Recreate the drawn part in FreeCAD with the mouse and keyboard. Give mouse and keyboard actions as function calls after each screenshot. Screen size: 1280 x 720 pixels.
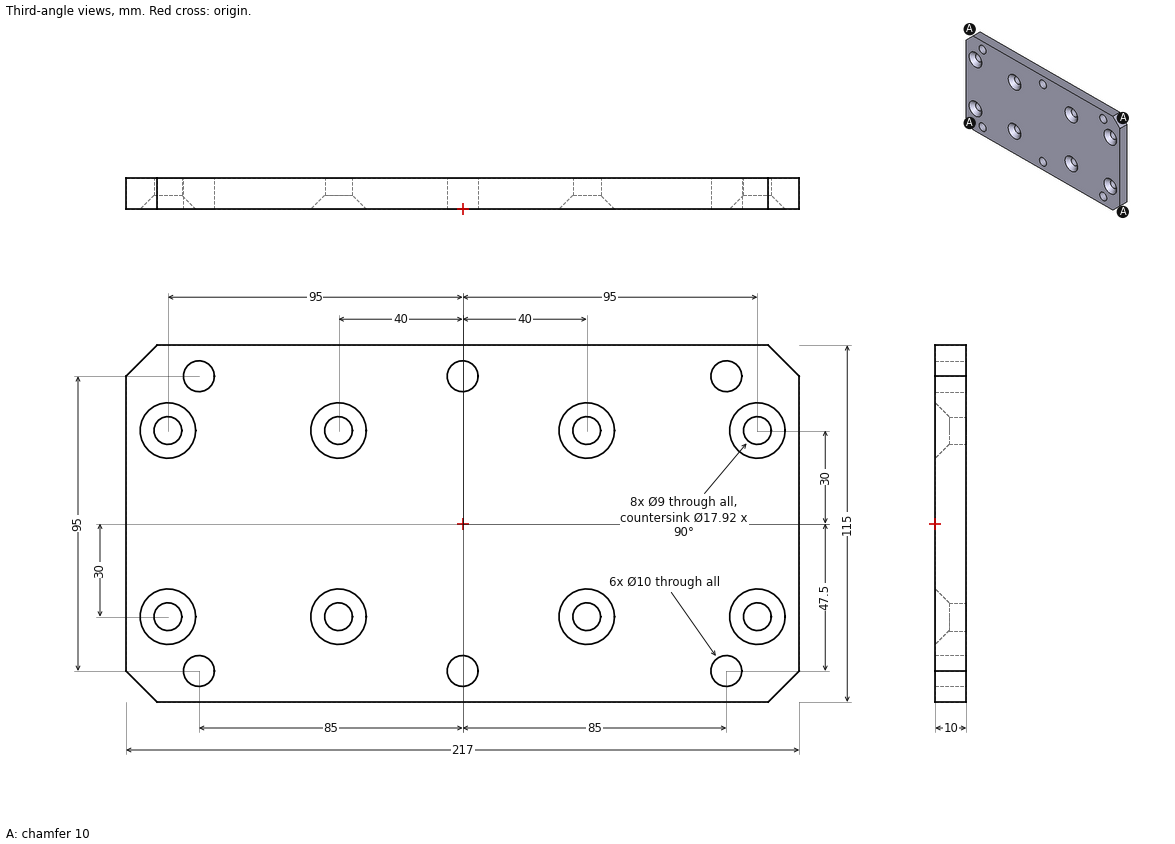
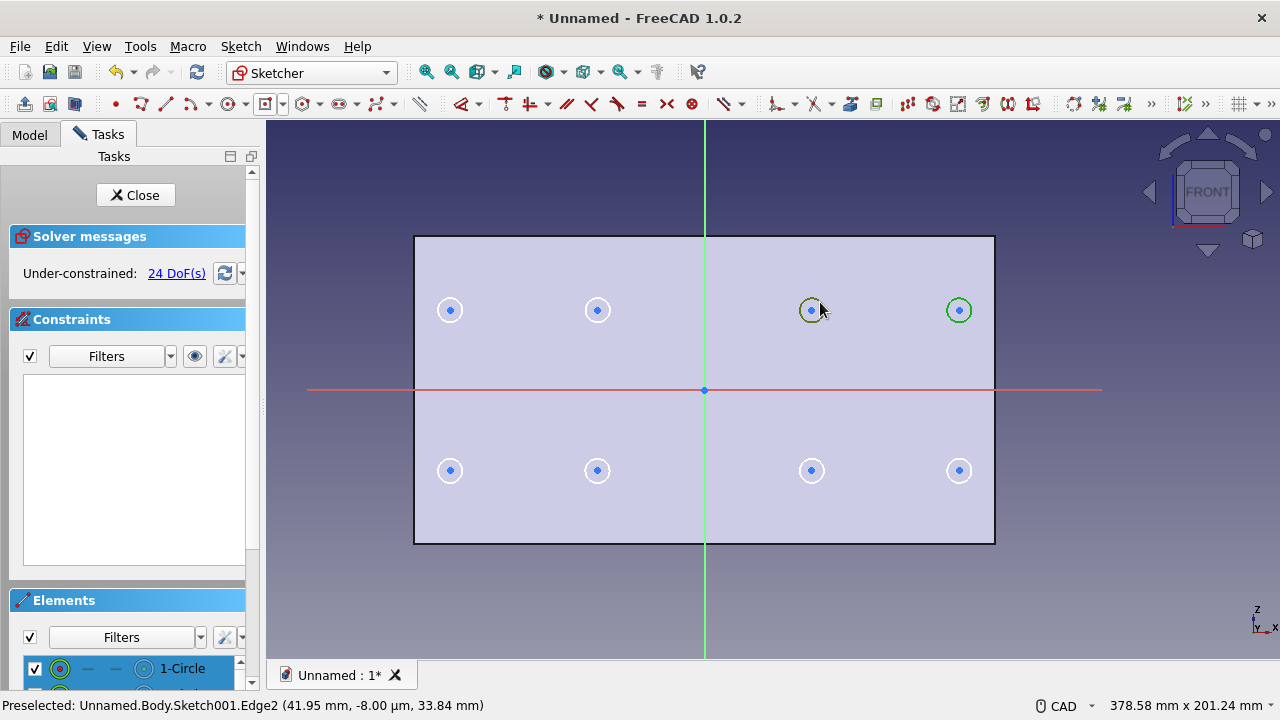
click(606, 302)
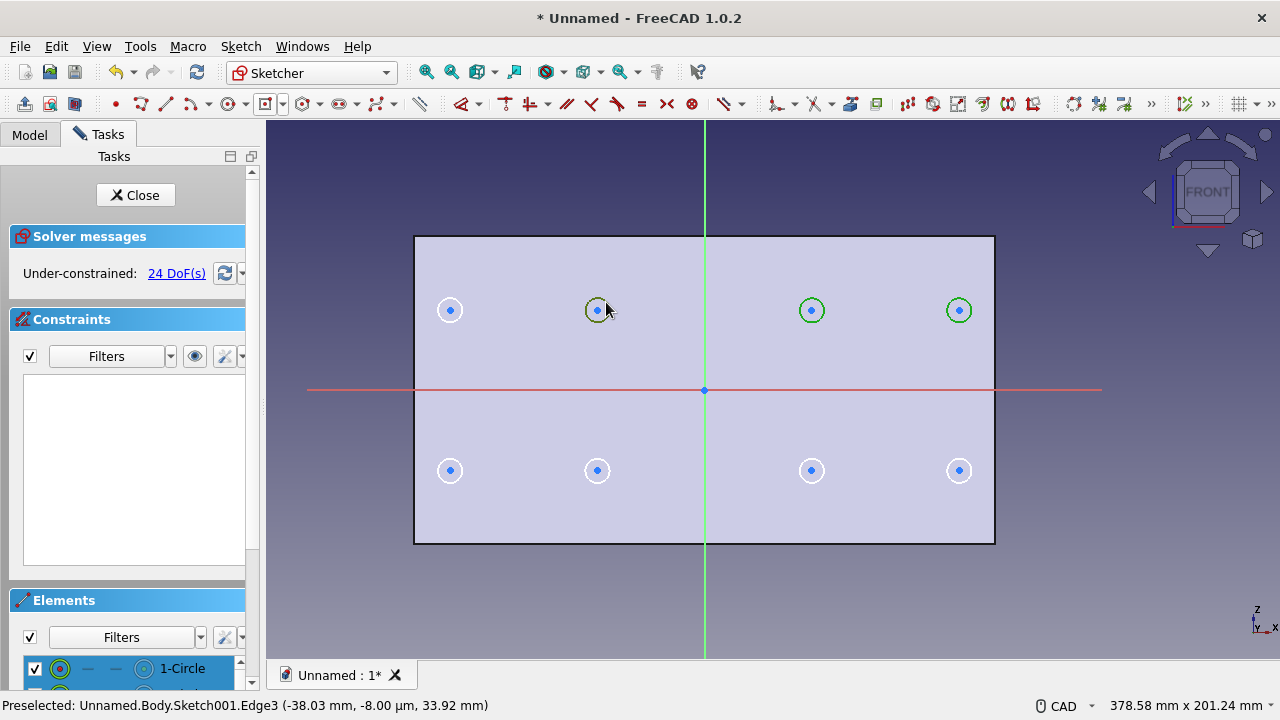
click(459, 302)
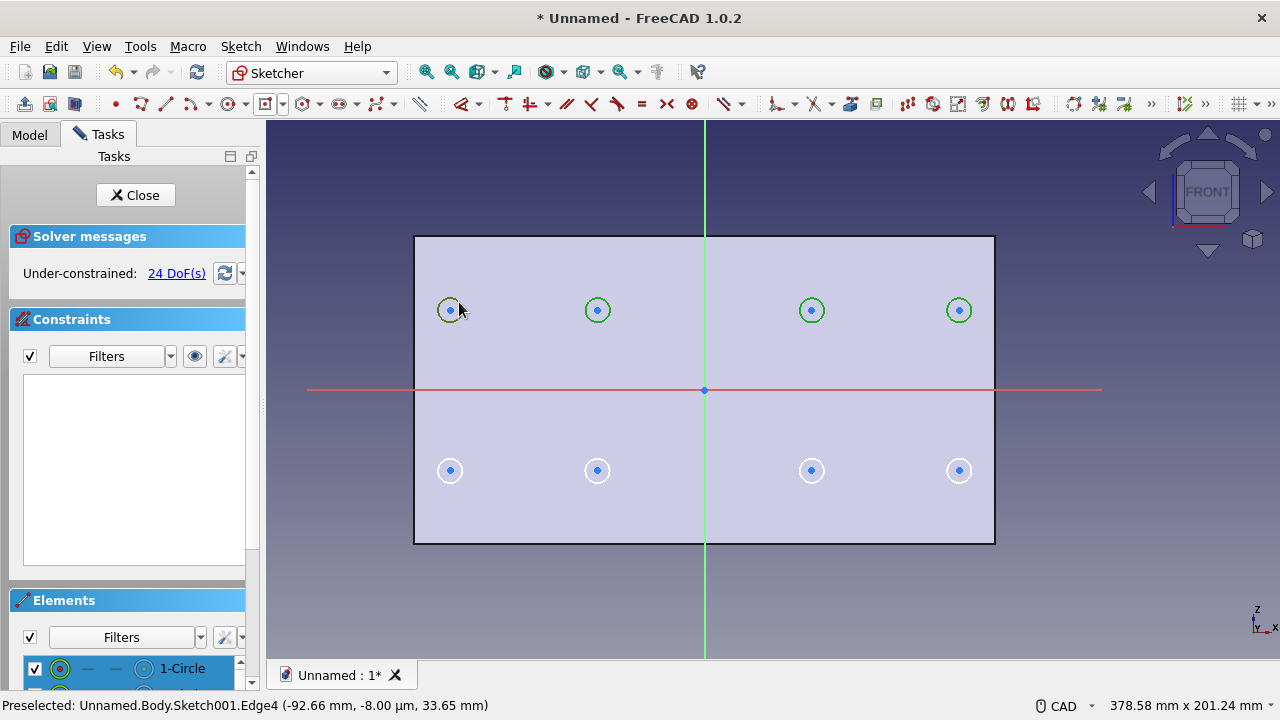
click(459, 462)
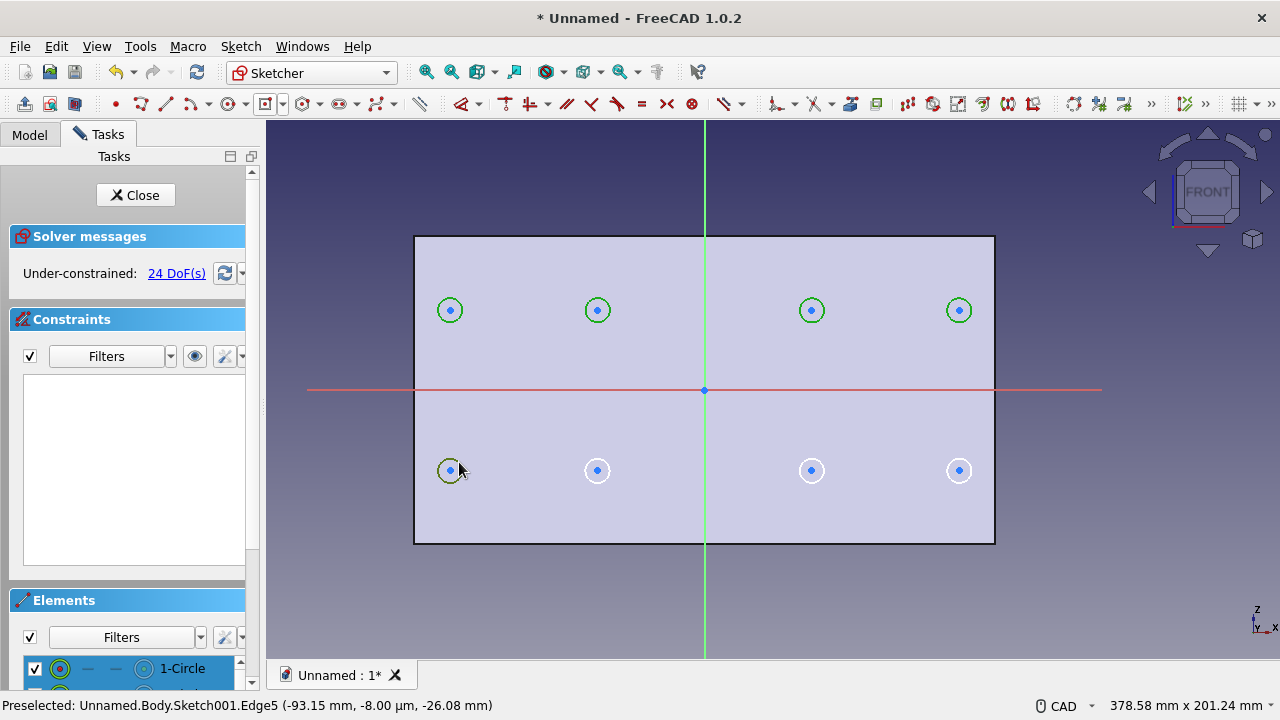
click(606, 462)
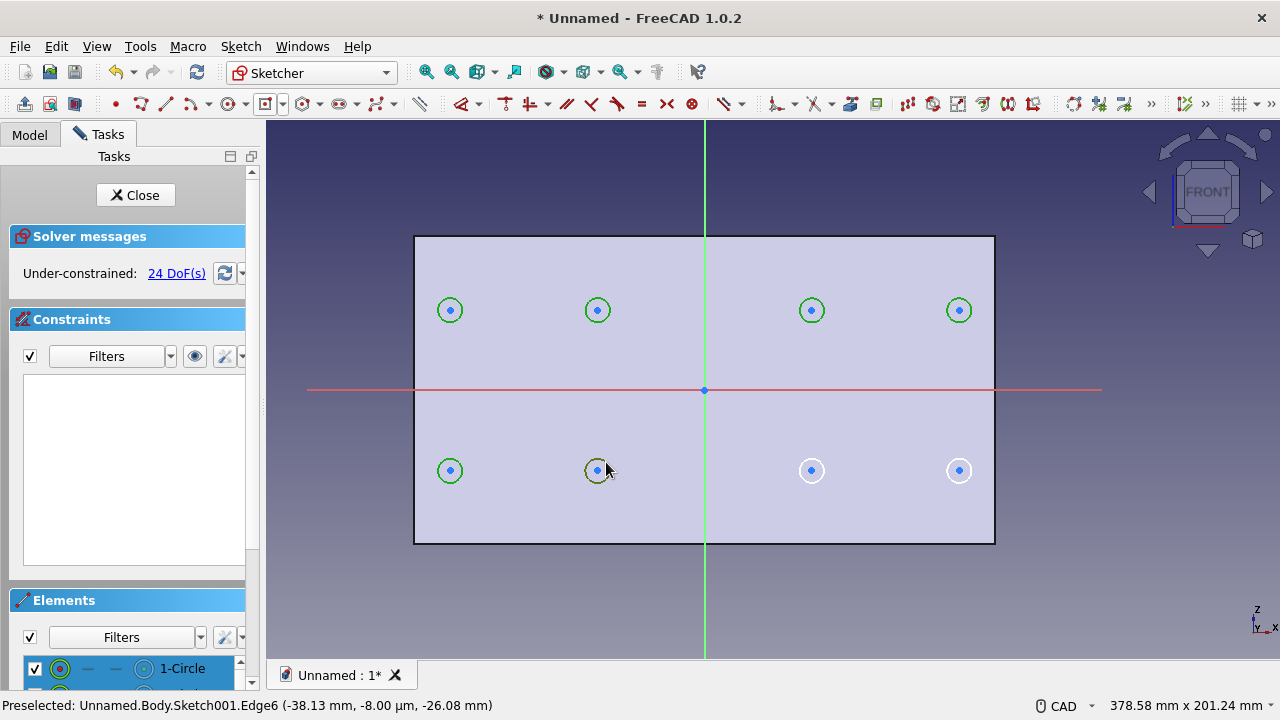
click(820, 462)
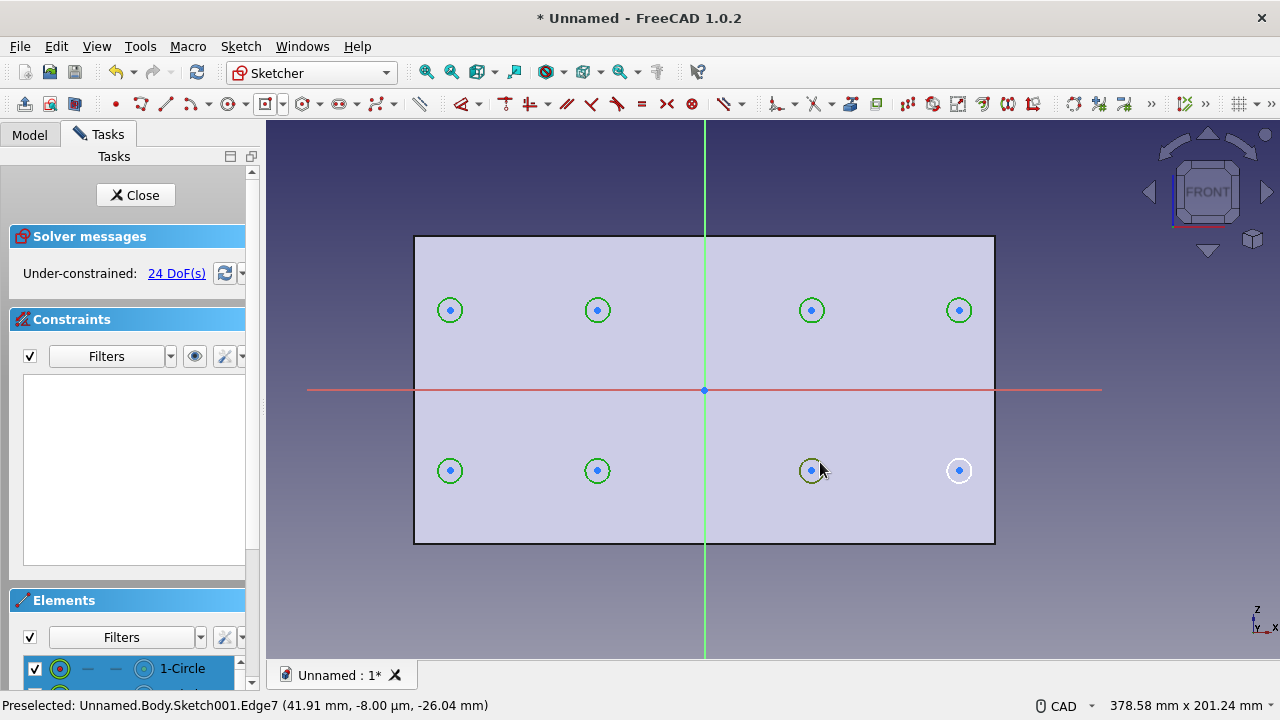
click(968, 462)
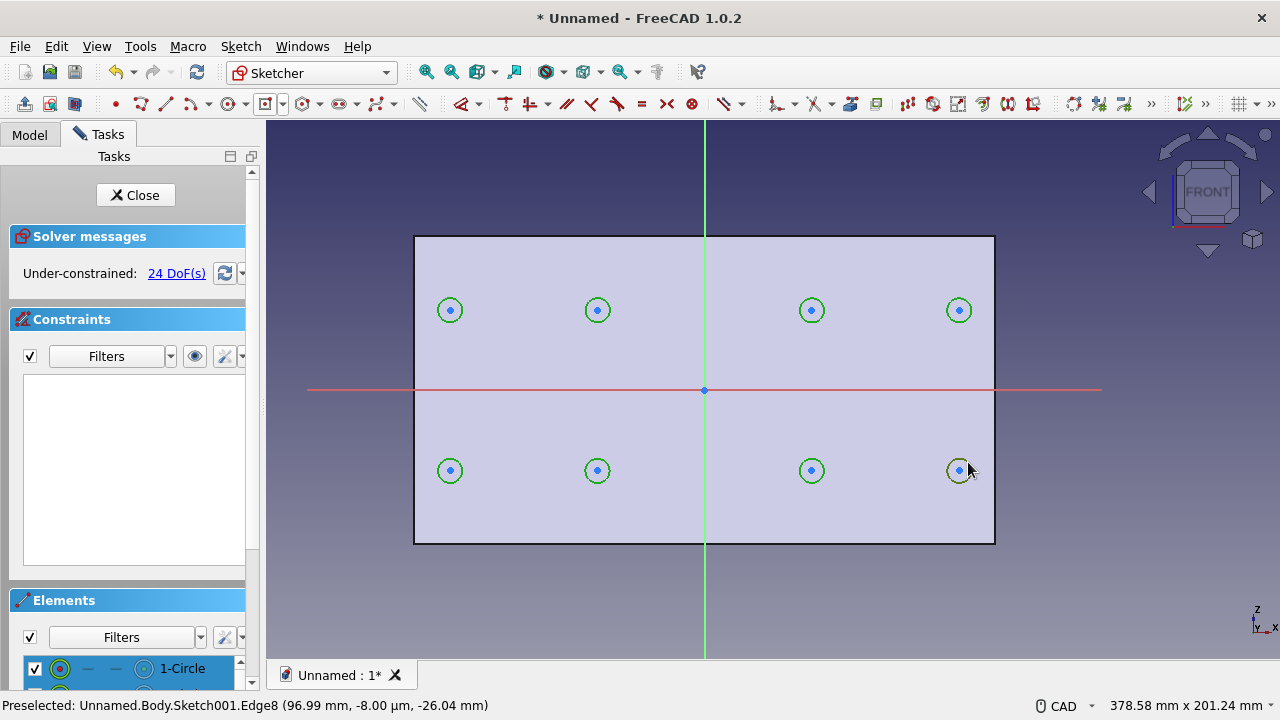
click(642, 104)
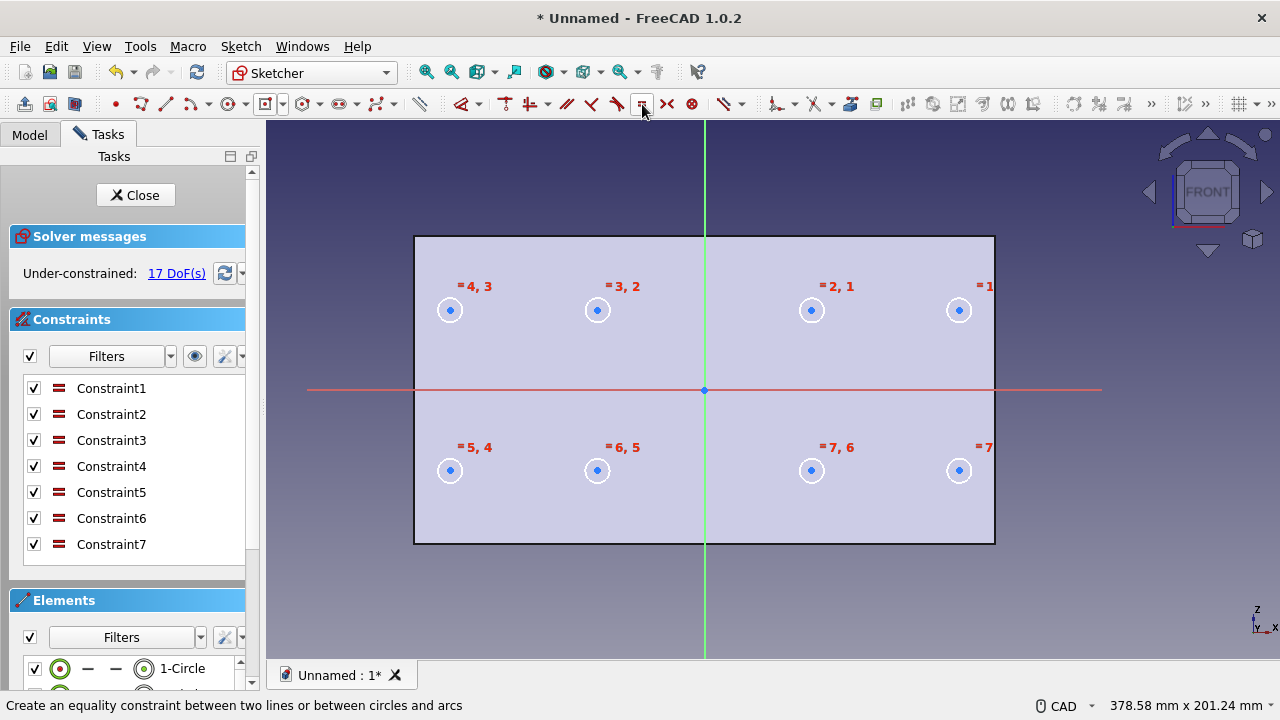
click(460, 104)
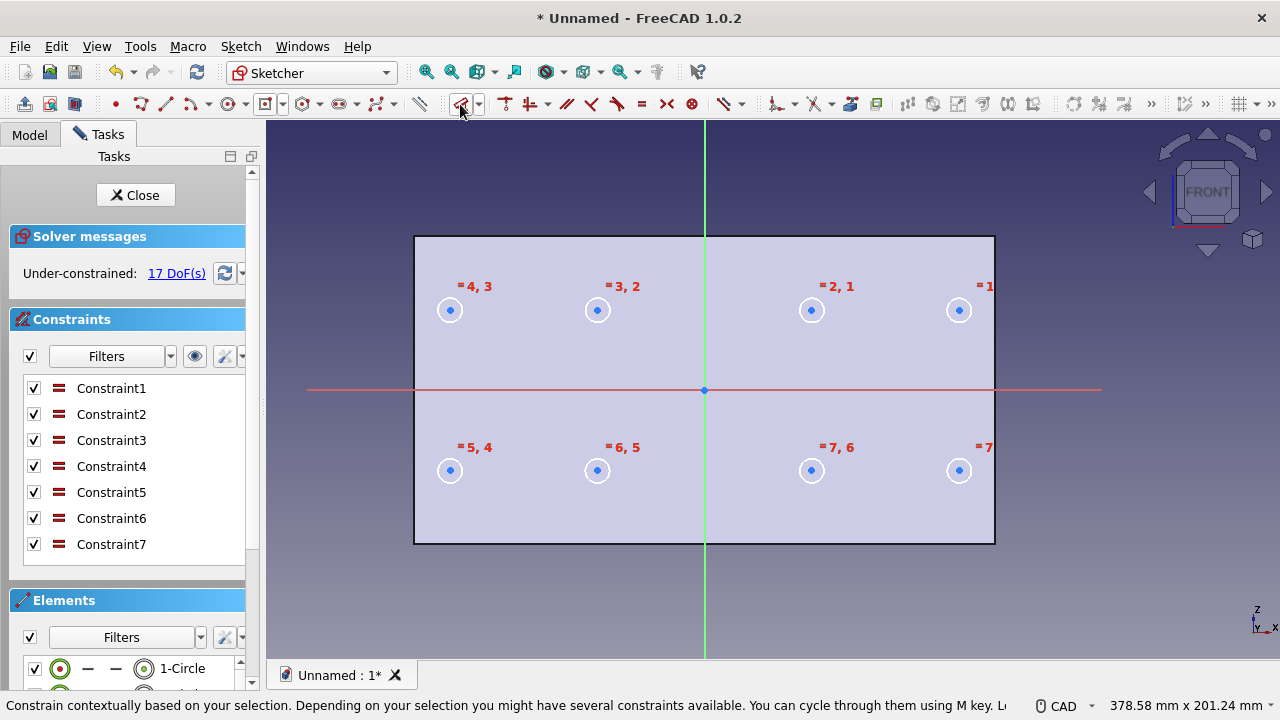
scroll(968, 302, up, 3)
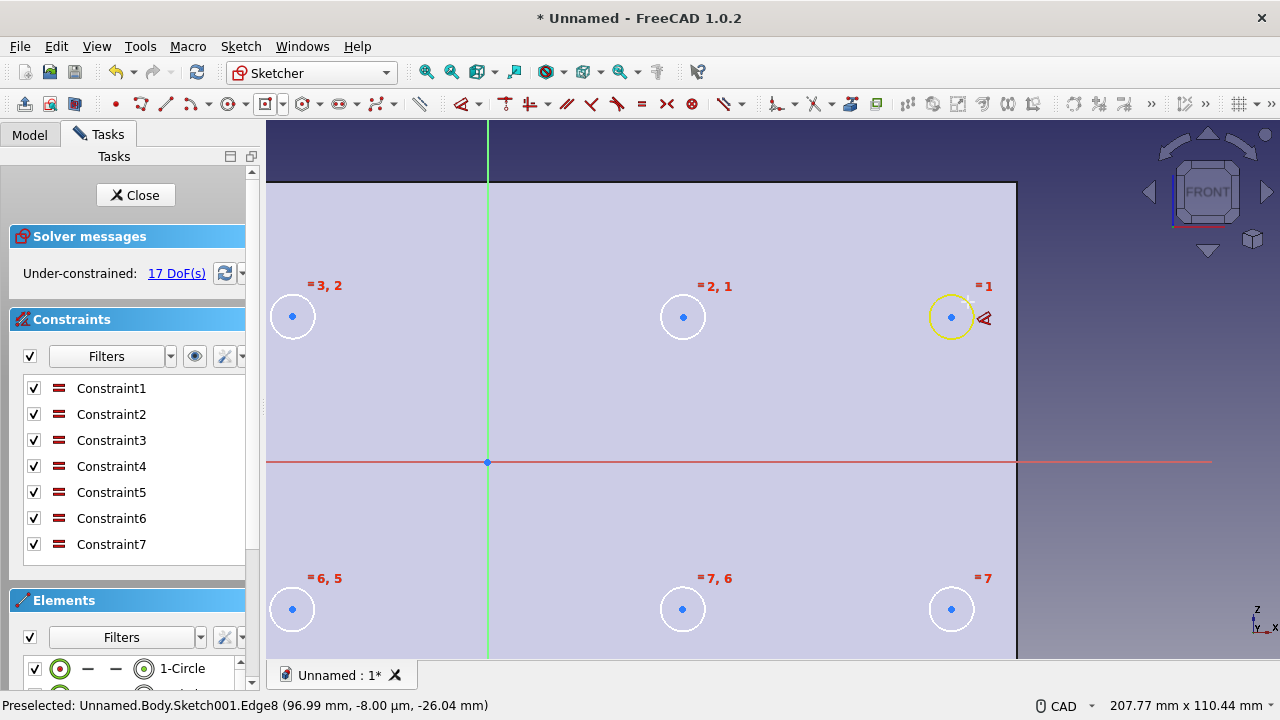
click(967, 301)
click(989, 278)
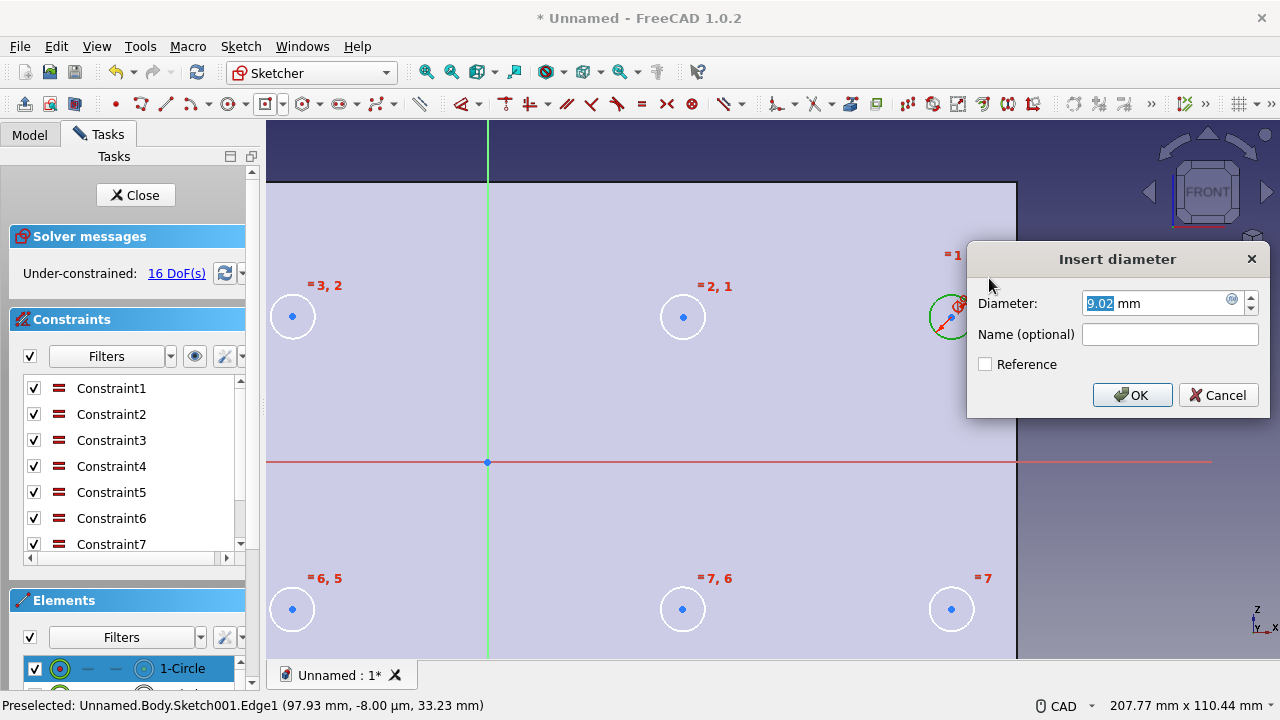
text(9)
key(Return)